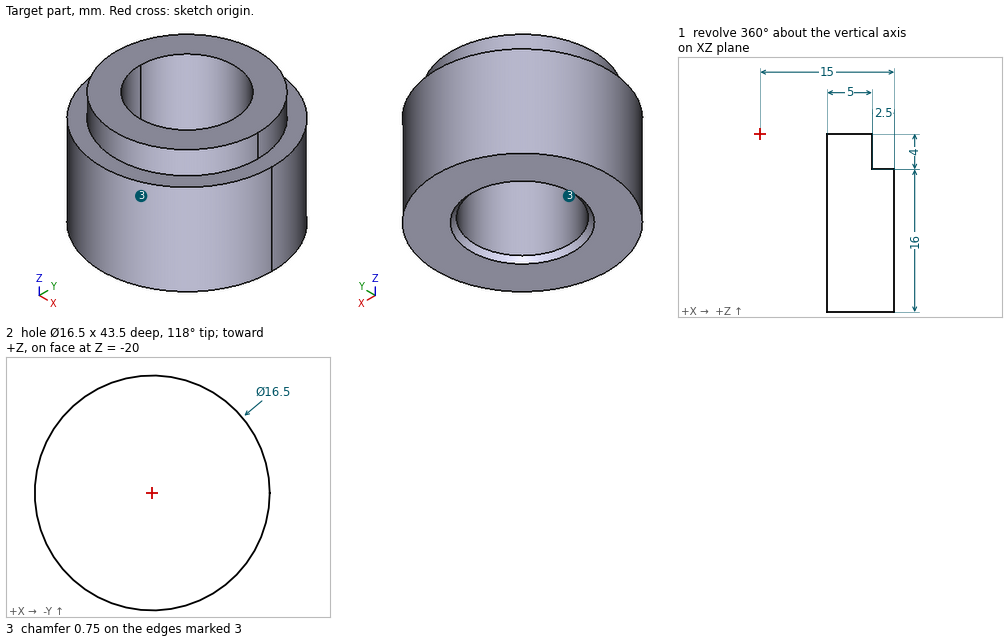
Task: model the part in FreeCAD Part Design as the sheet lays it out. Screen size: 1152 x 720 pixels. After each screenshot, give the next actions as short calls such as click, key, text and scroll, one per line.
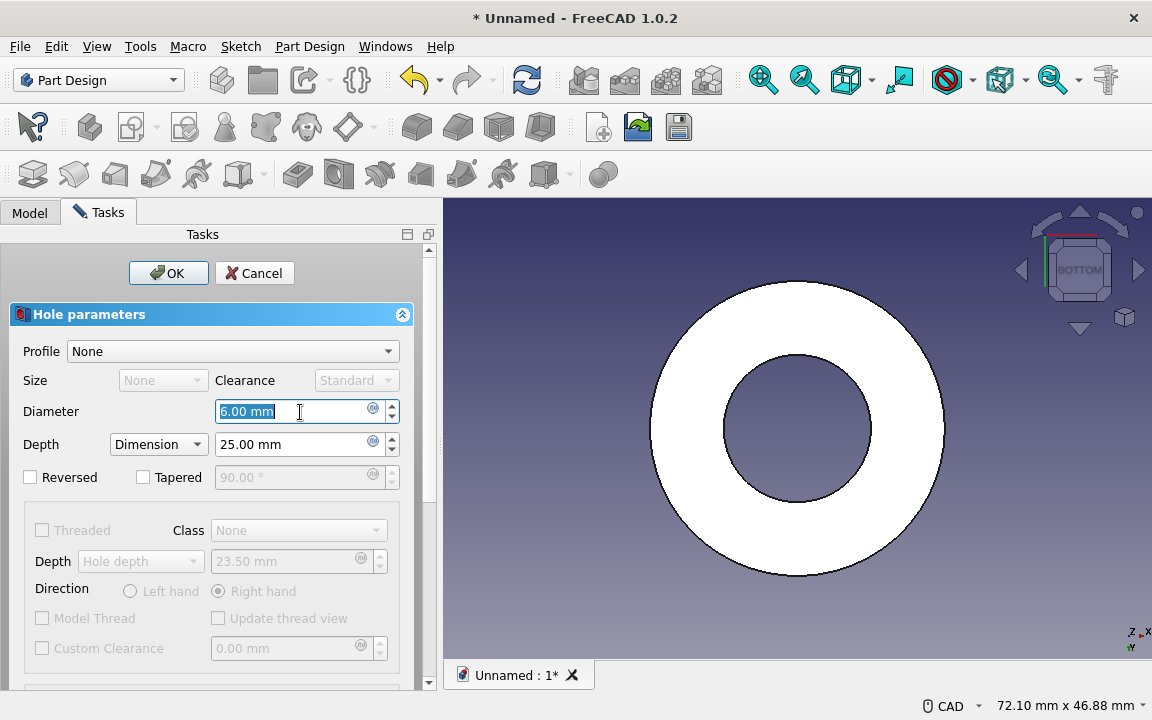
text(16.5)
key(Tab)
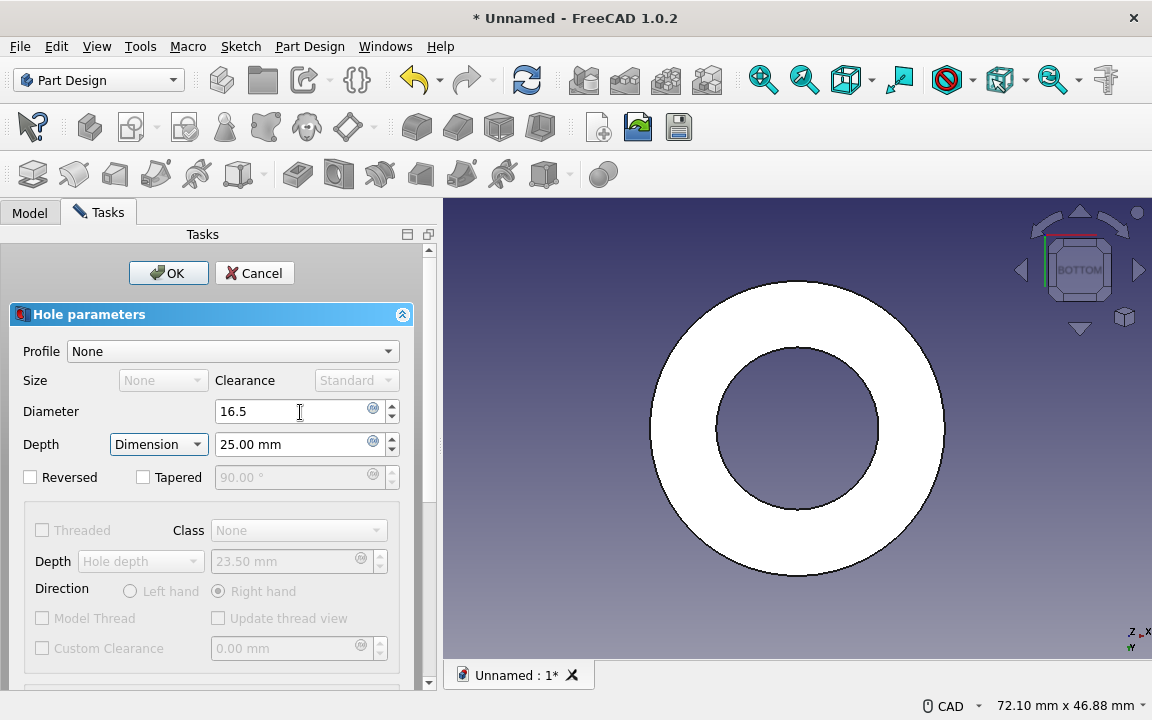
triple_click(300, 444)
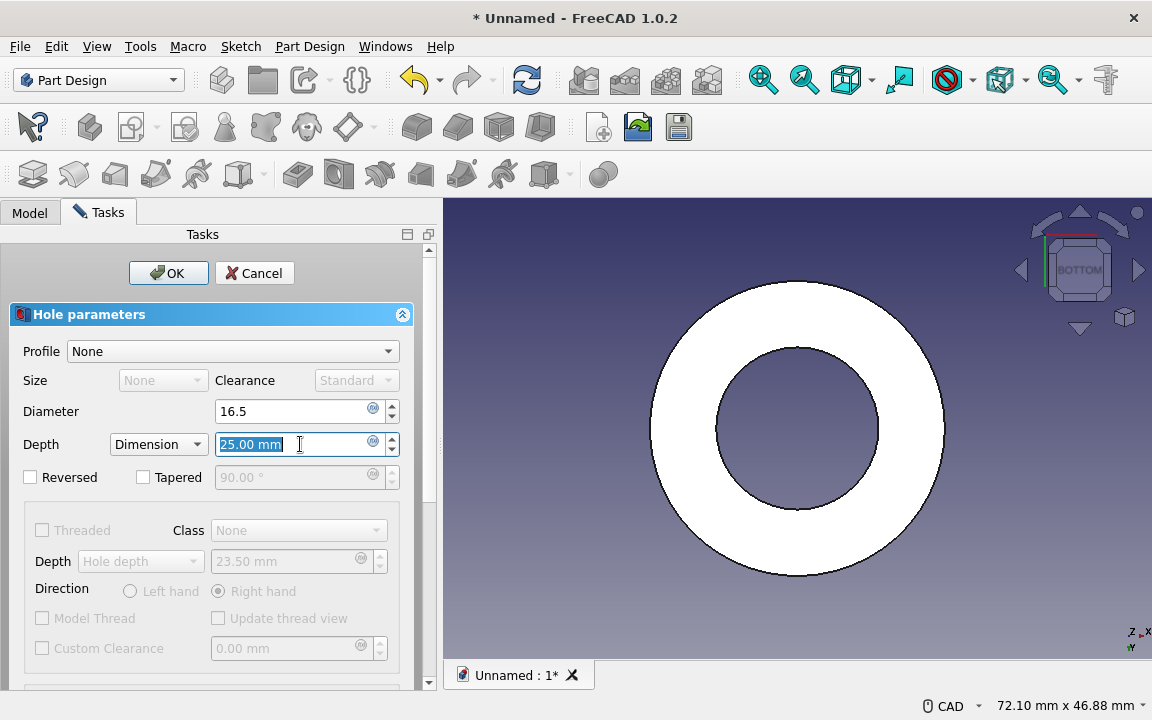
text(43.5)
key(Tab)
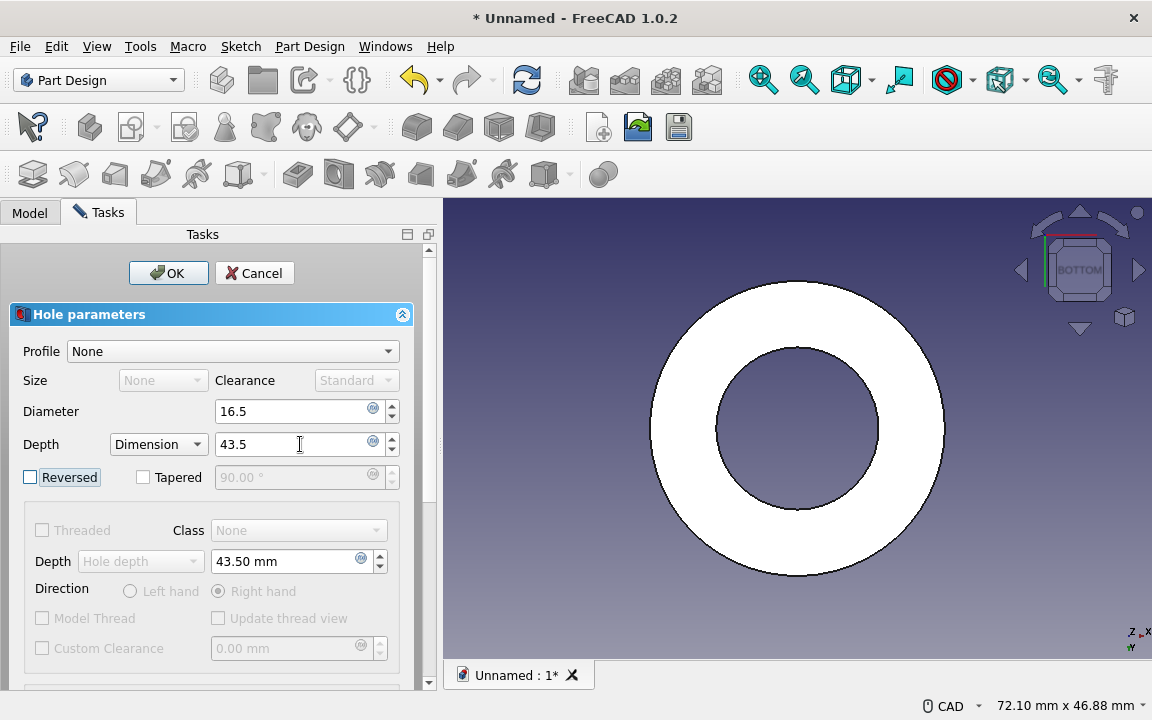
click(169, 273)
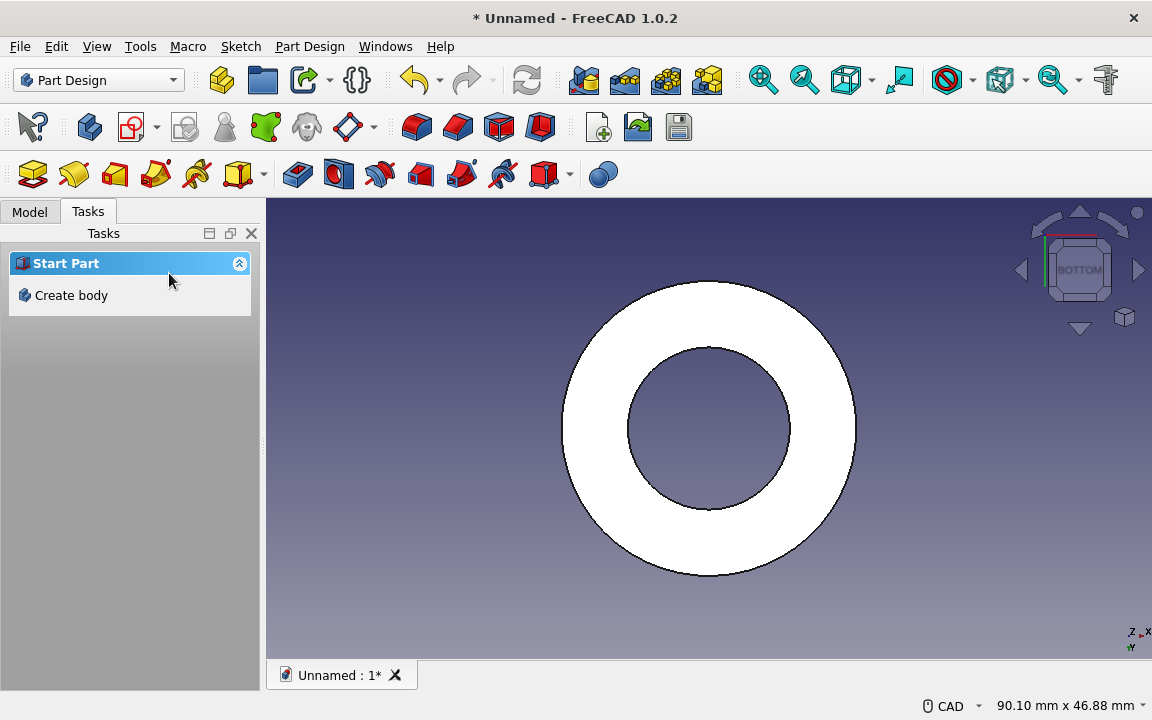
click(775, 475)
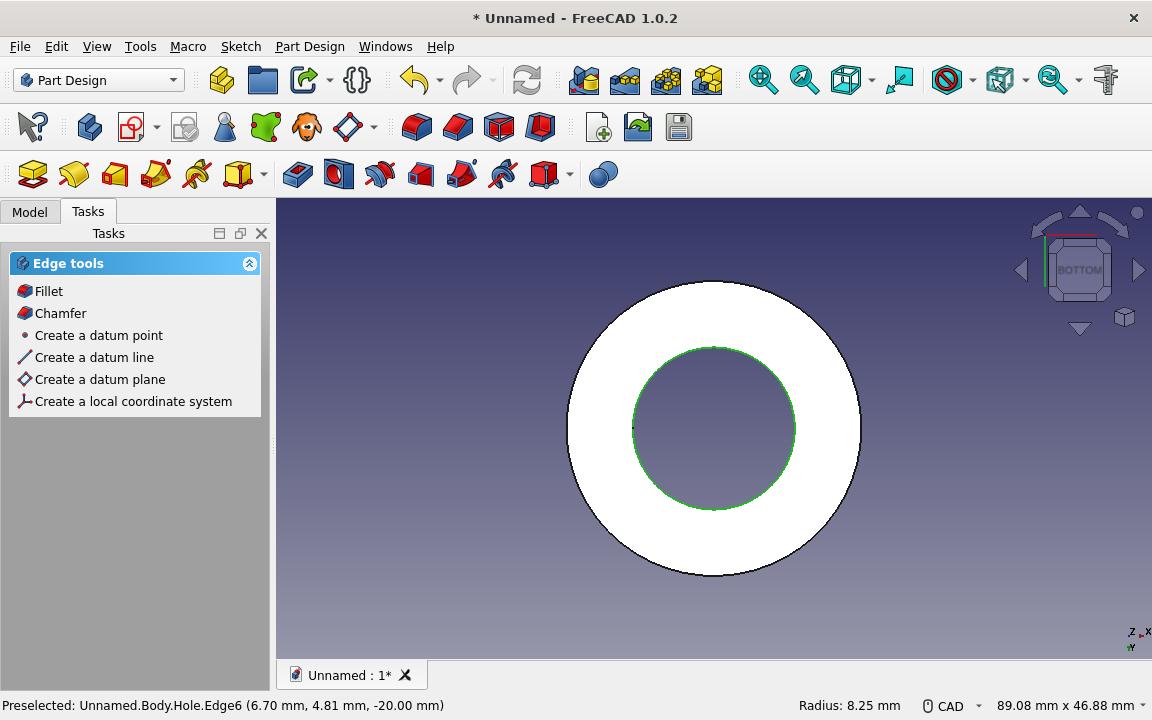
click(458, 128)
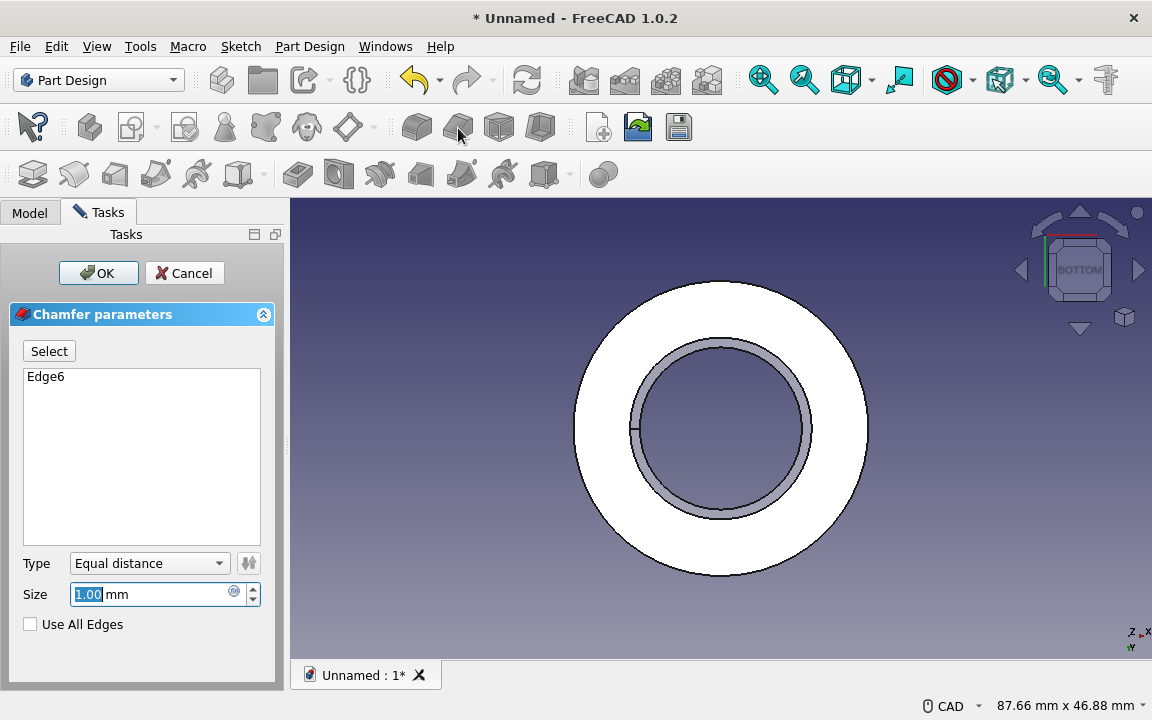
text(0.75)
key(Tab)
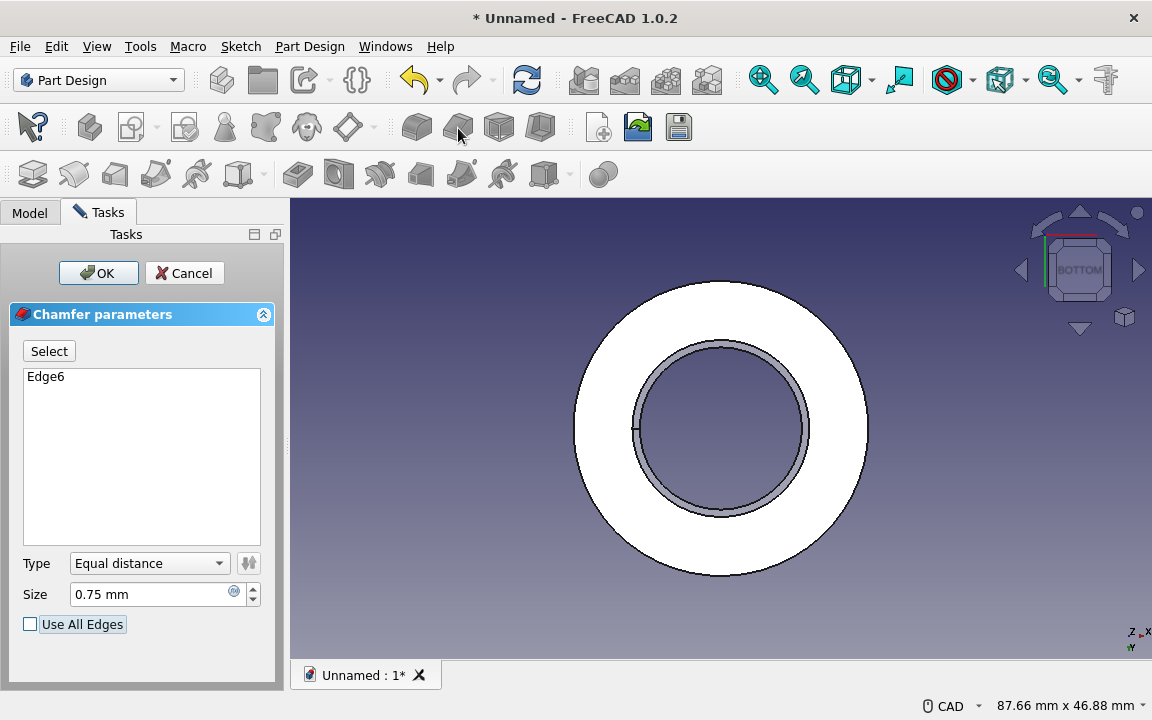
click(99, 273)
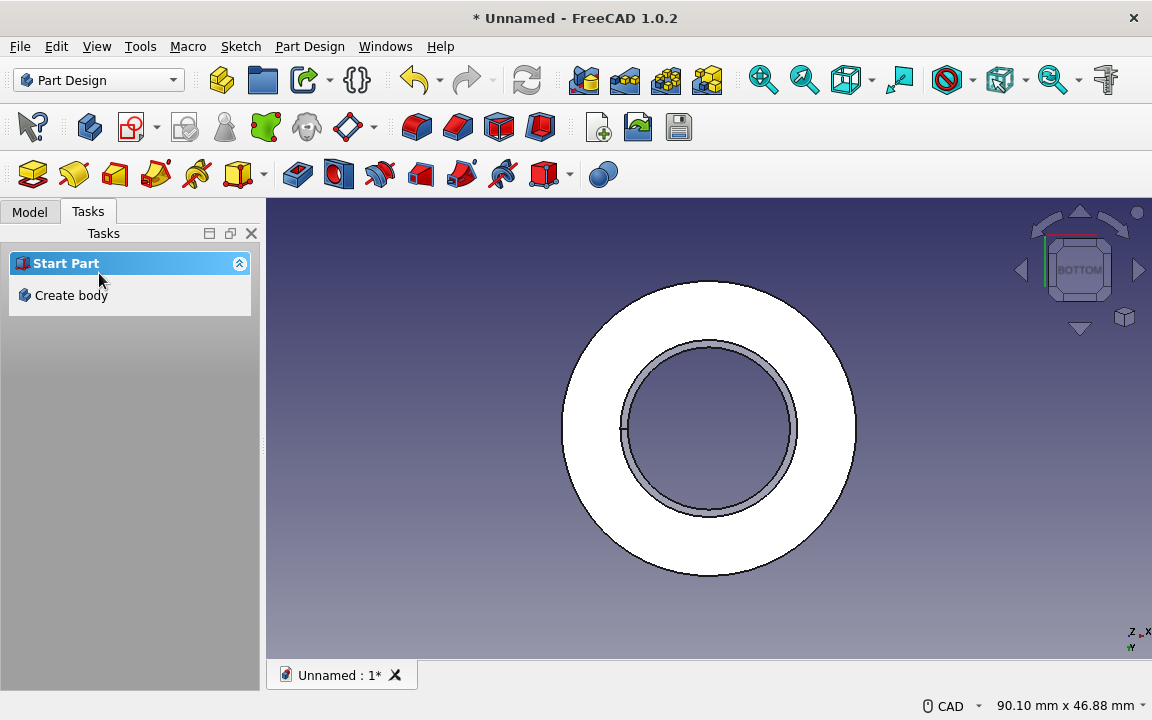
key(0)